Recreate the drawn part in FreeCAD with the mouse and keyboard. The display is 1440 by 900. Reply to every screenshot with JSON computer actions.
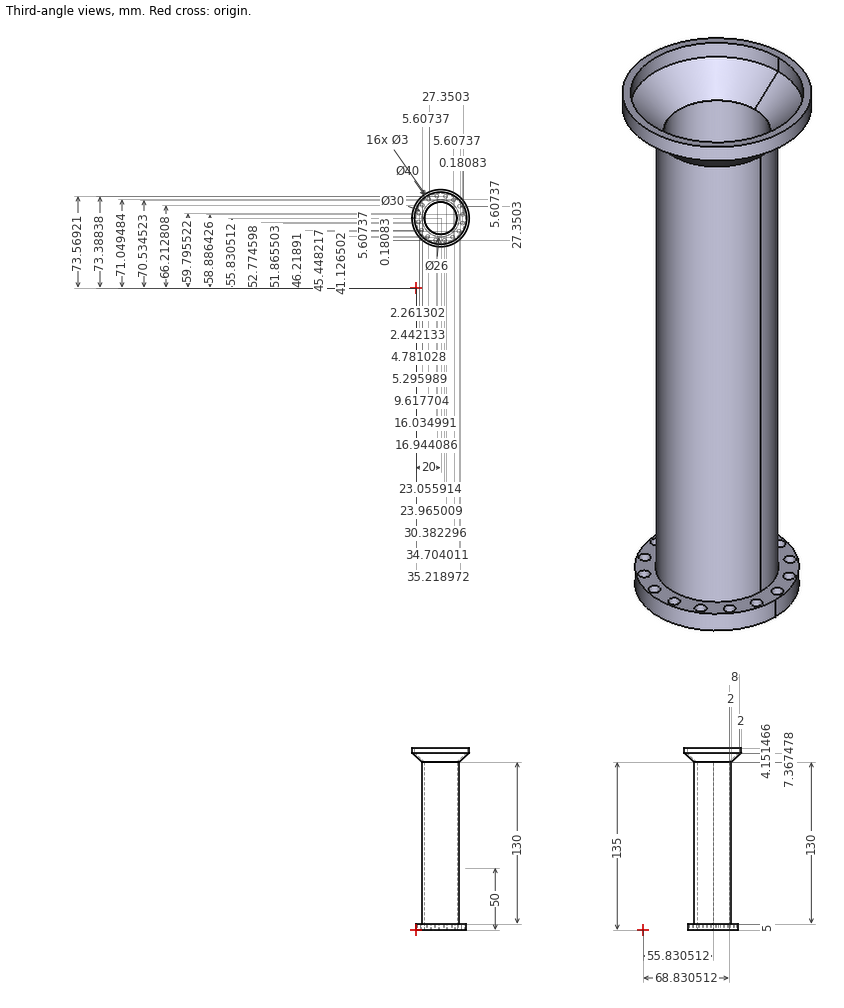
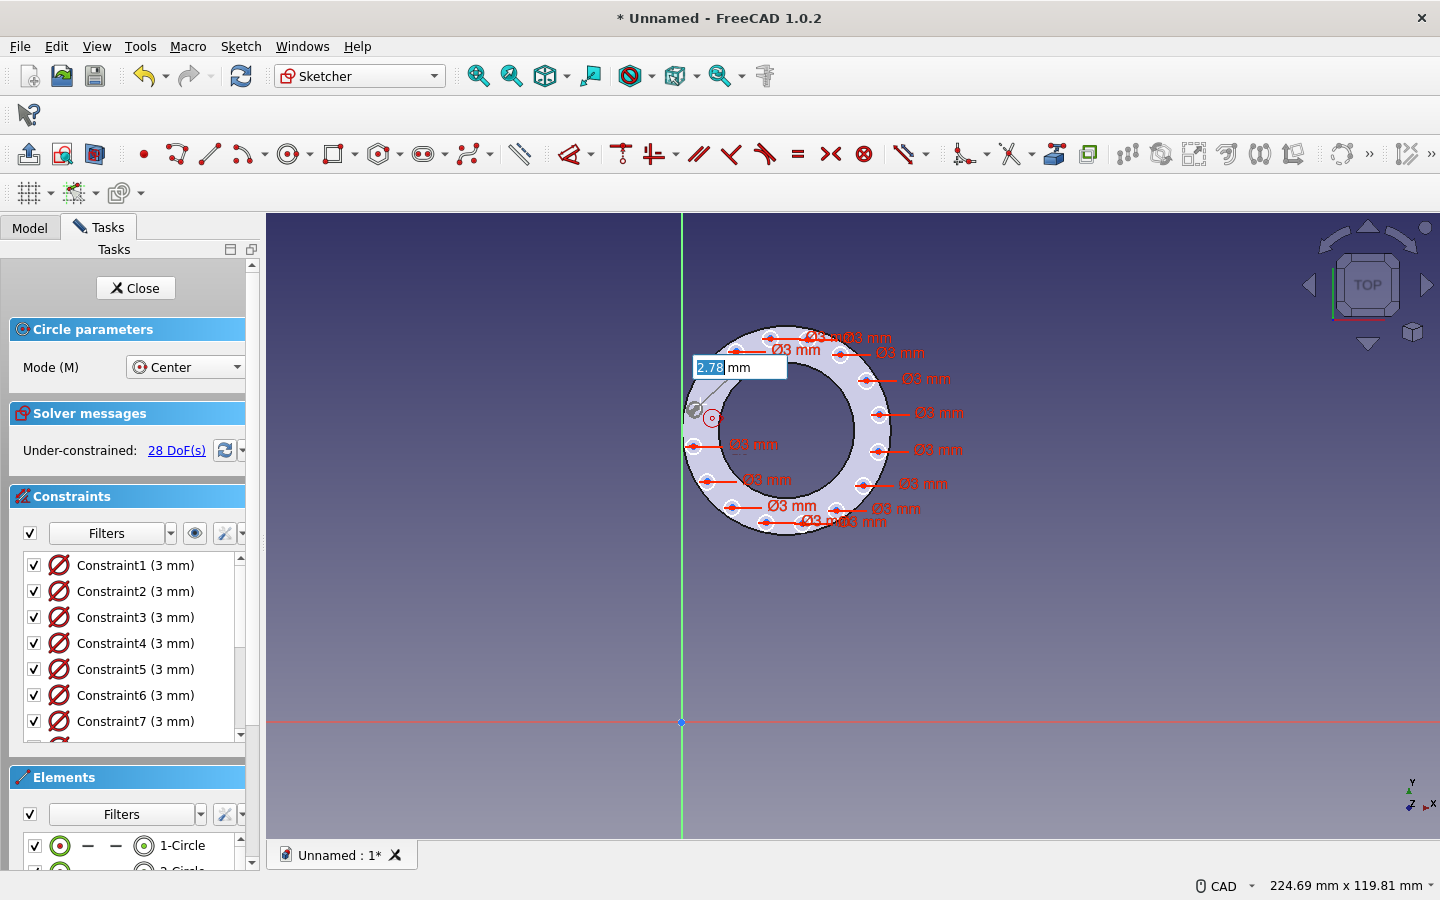
{"action": "type", "text": "3"}
{"action": "key", "text": "Return"}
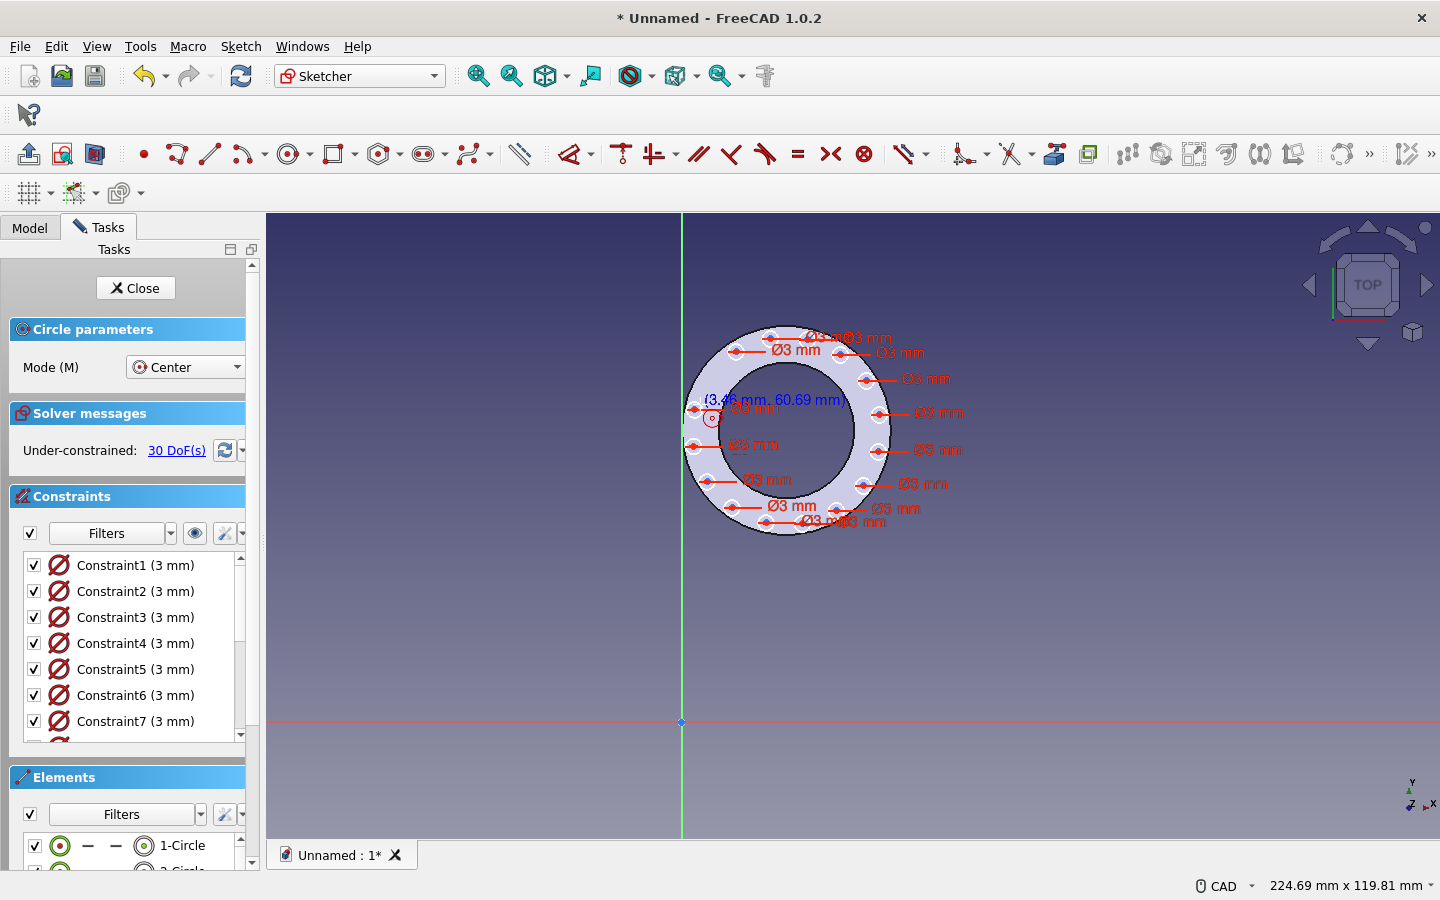
{"action": "scroll", "coordinate": [710, 376], "scroll_direction": "up", "scroll_amount": 6}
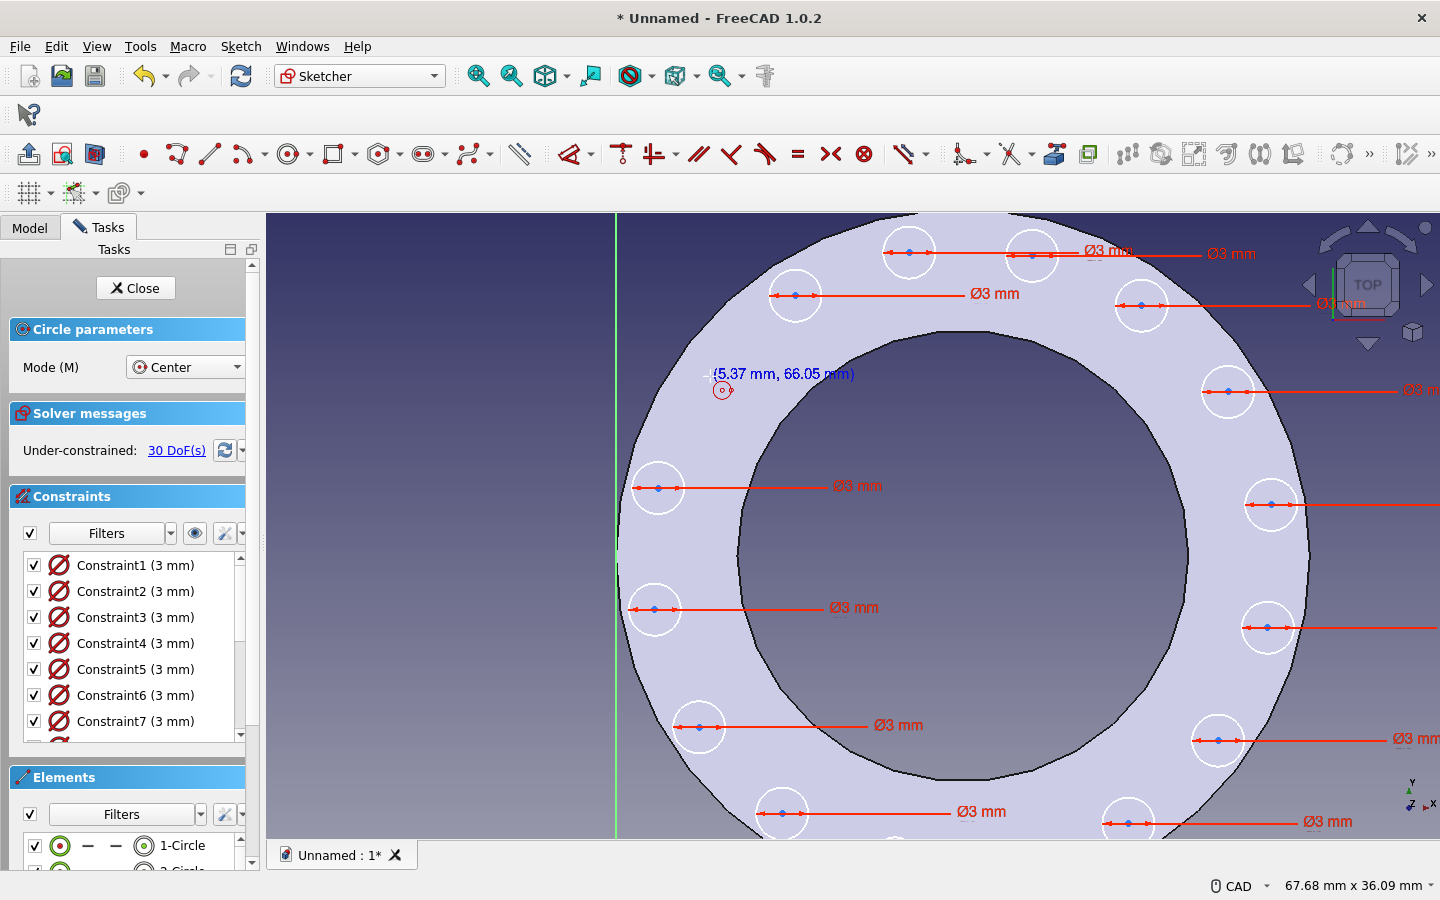
{"action": "scroll", "coordinate": [710, 376], "scroll_direction": "down", "scroll_amount": 6}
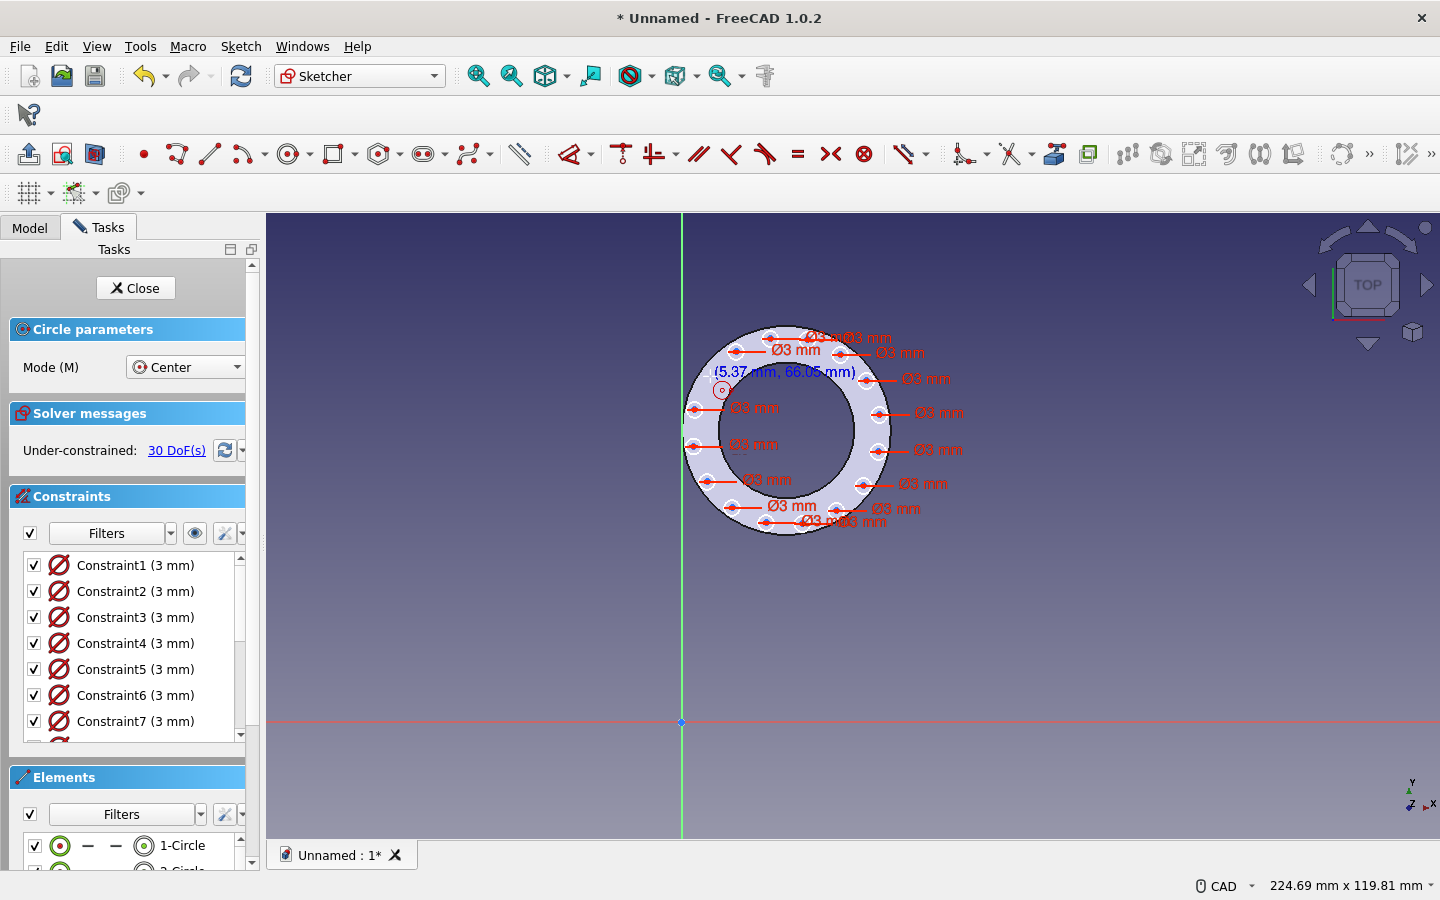
{"action": "left_click", "coordinate": [710, 376]}
{"action": "mouse_move", "coordinate": [715, 371]}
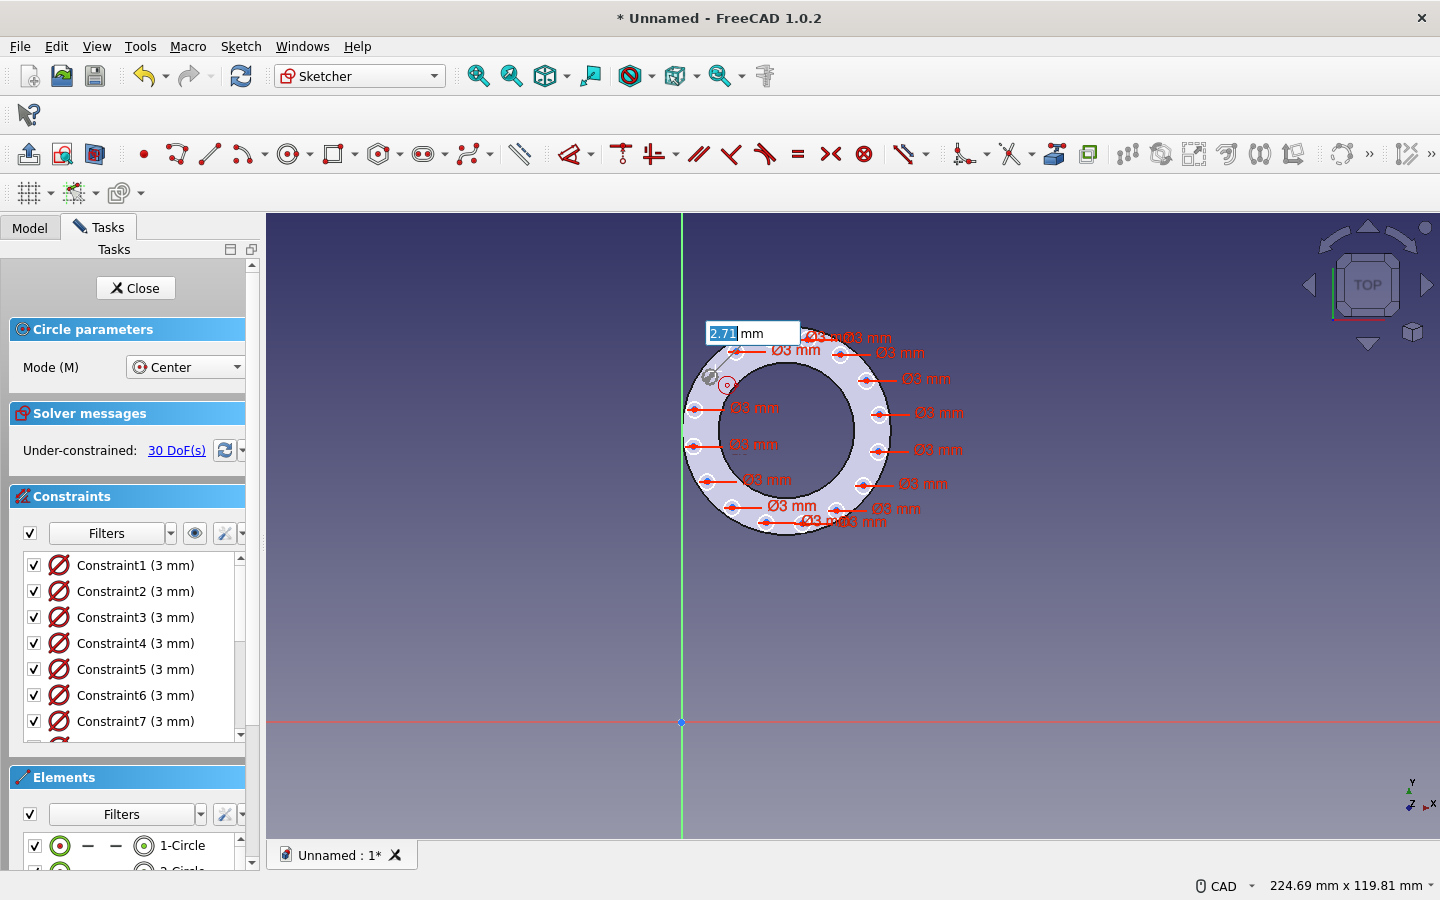
{"action": "type", "text": "3"}
{"action": "key", "text": "Return"}
{"action": "key", "text": "Escape"}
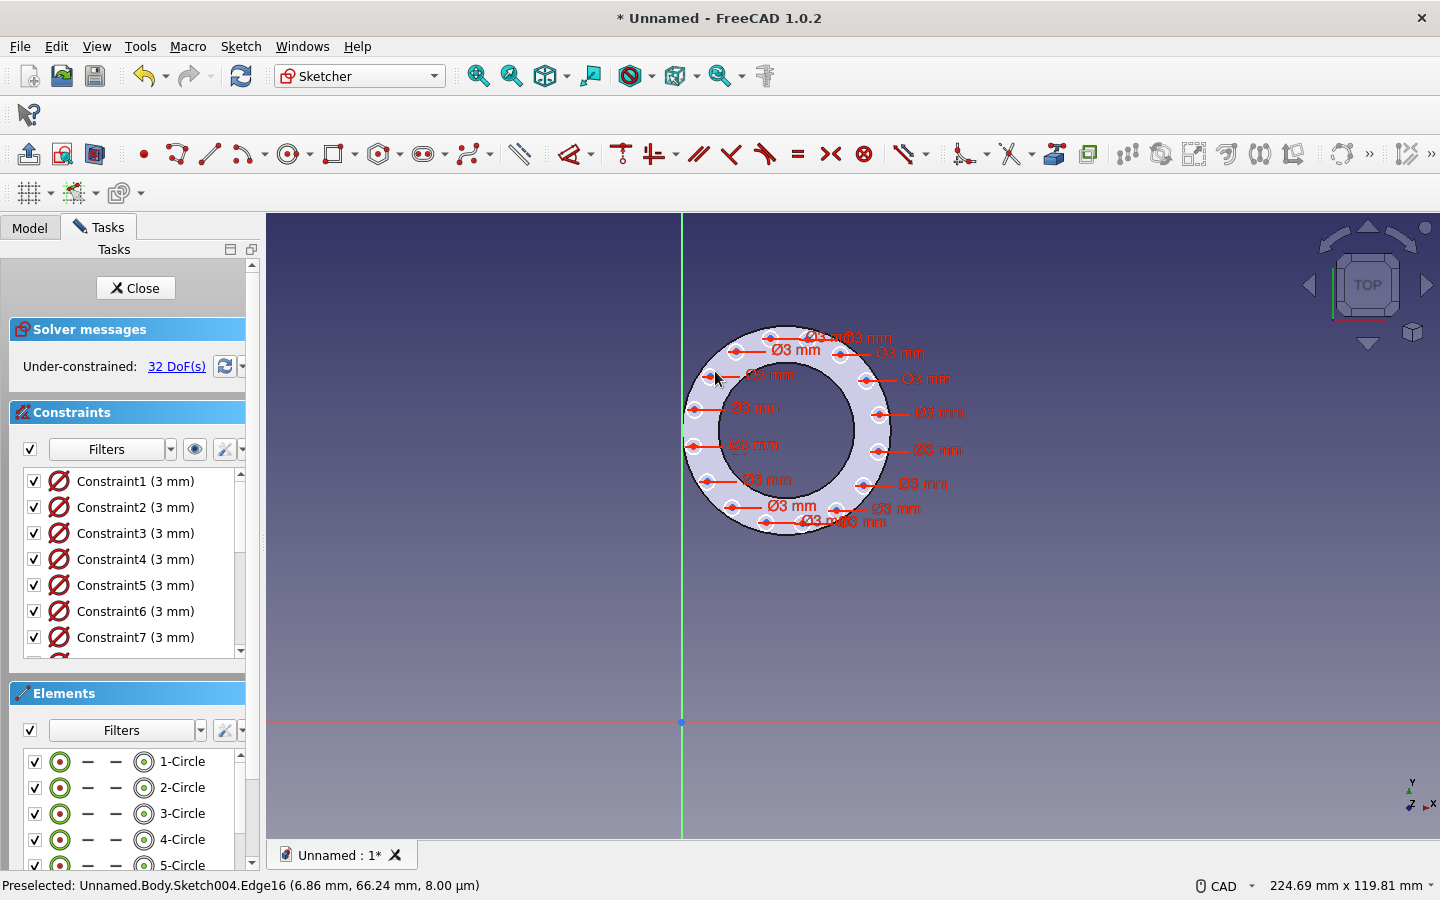
{"action": "left_click", "coordinate": [568, 154]}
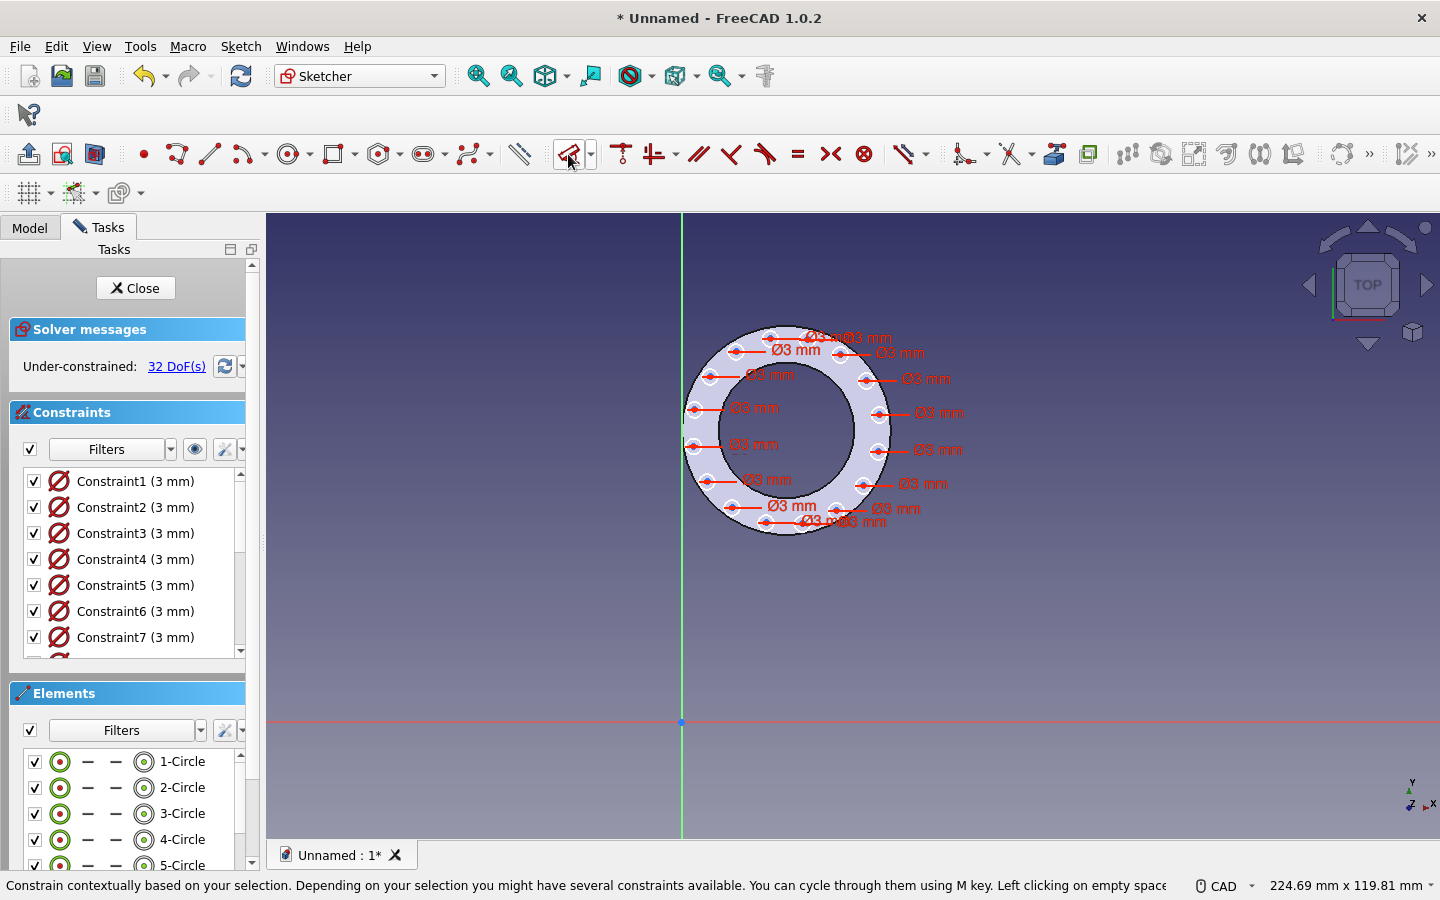
{"action": "left_click", "coordinate": [770, 339]}
{"action": "left_click", "coordinate": [648, 531]}